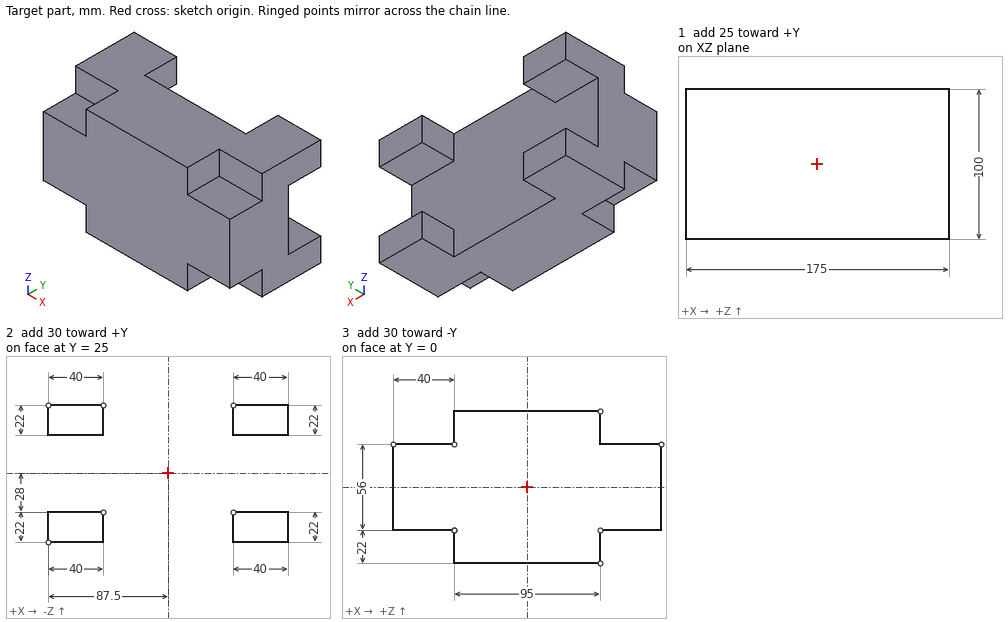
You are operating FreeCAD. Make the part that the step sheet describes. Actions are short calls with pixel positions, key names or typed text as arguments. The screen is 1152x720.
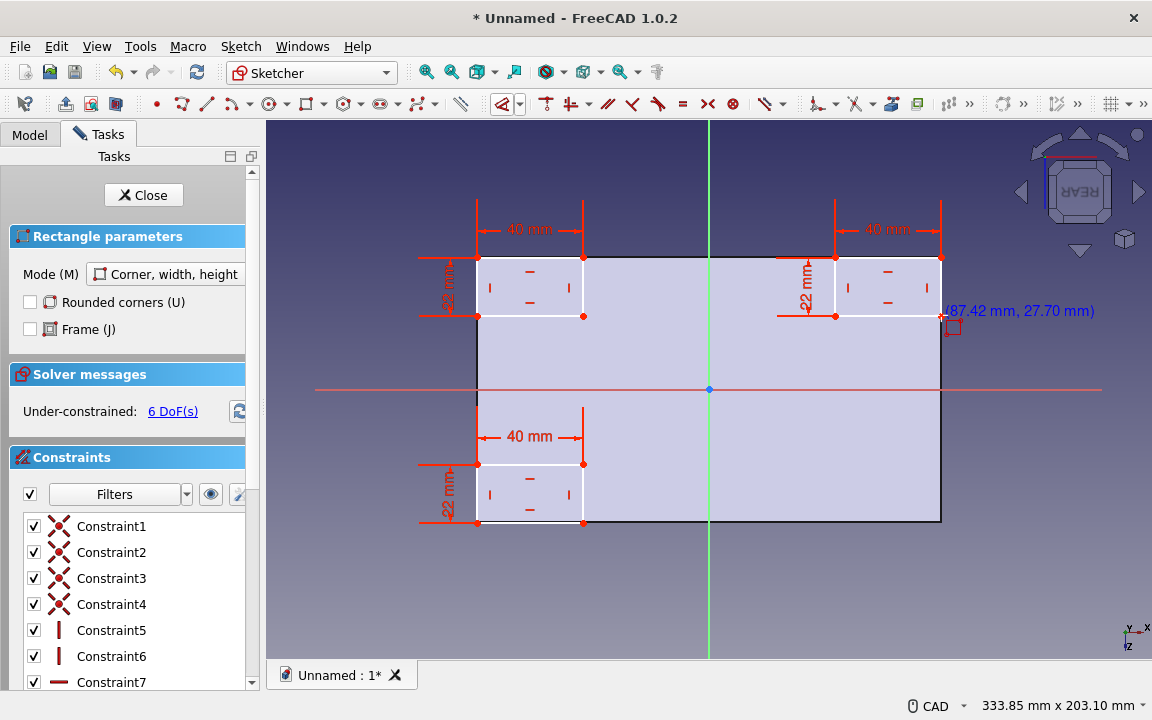
click(835, 464)
move(941, 522)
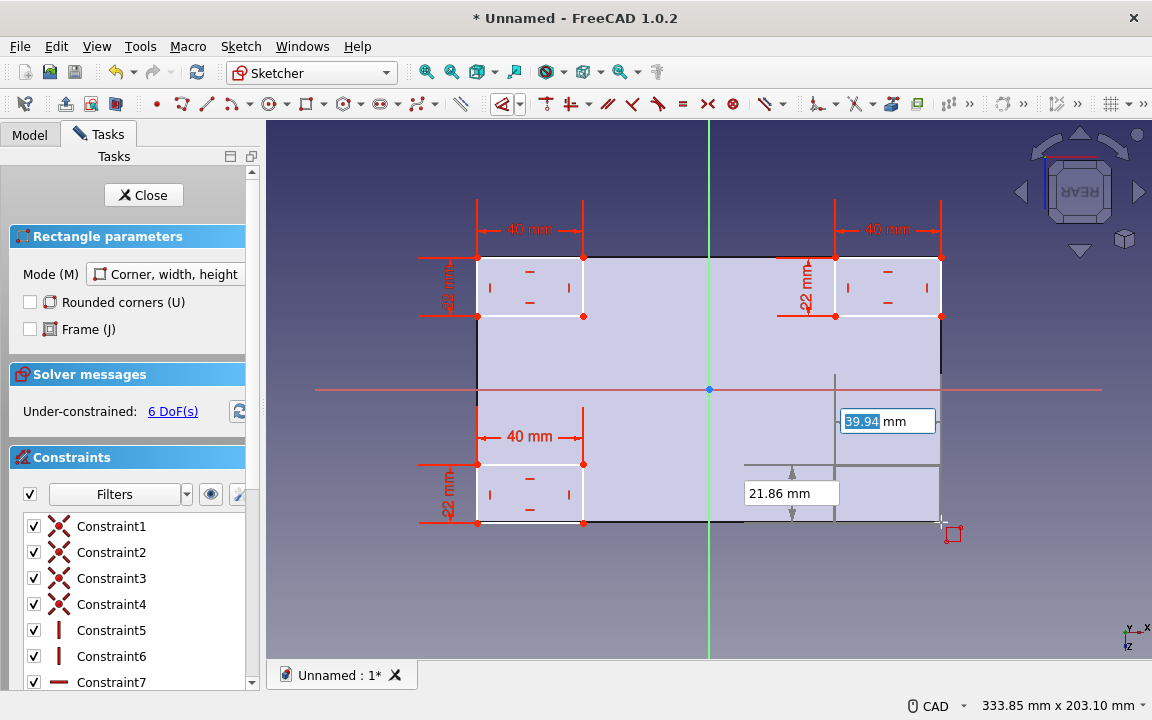
text(40)
key(Tab)
text(22)
key(Return)
key(Escape)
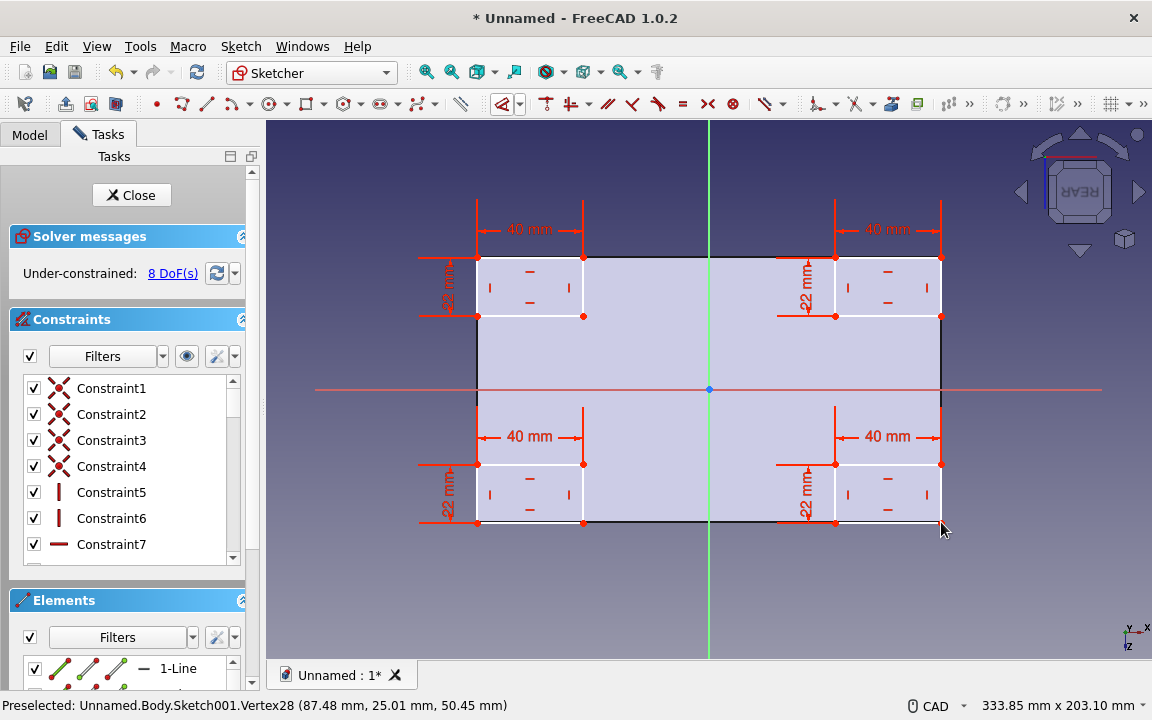
click(477, 523)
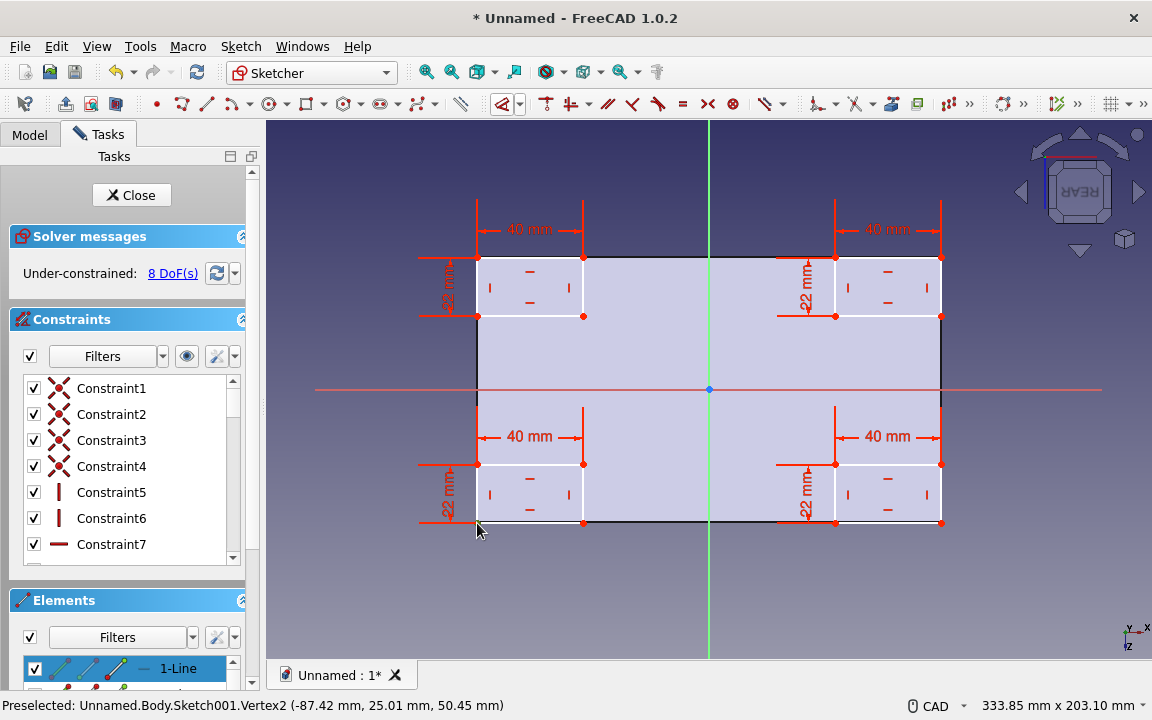
click(477, 258)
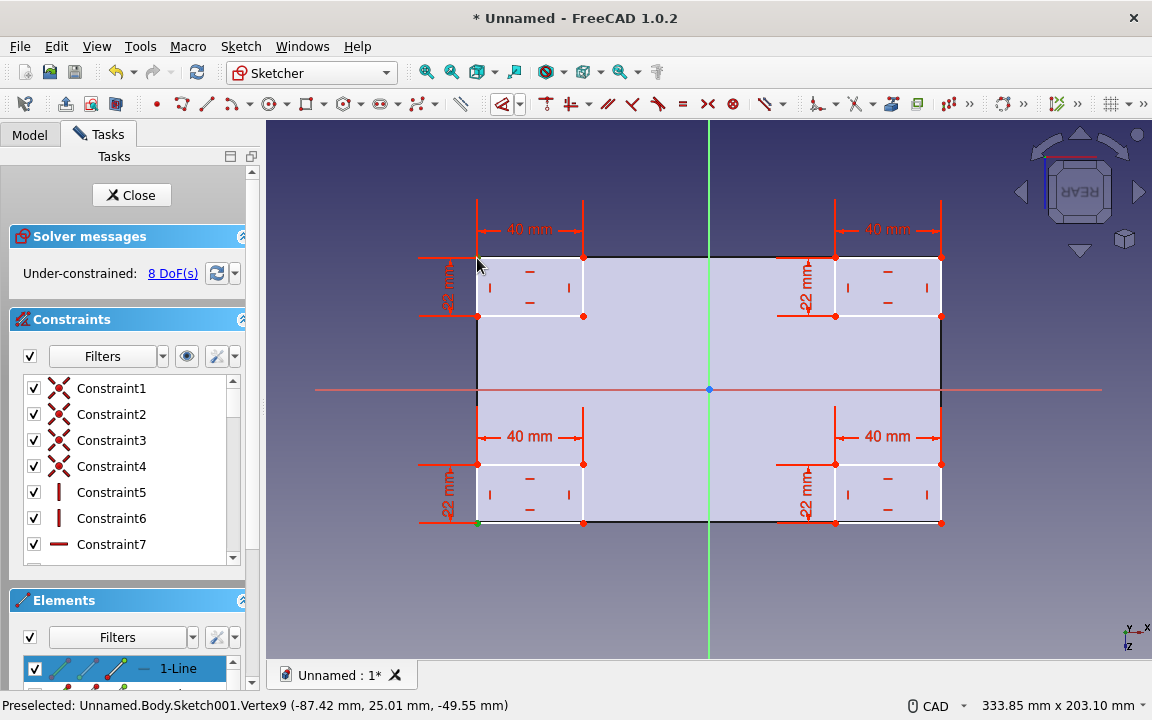
click(343, 390)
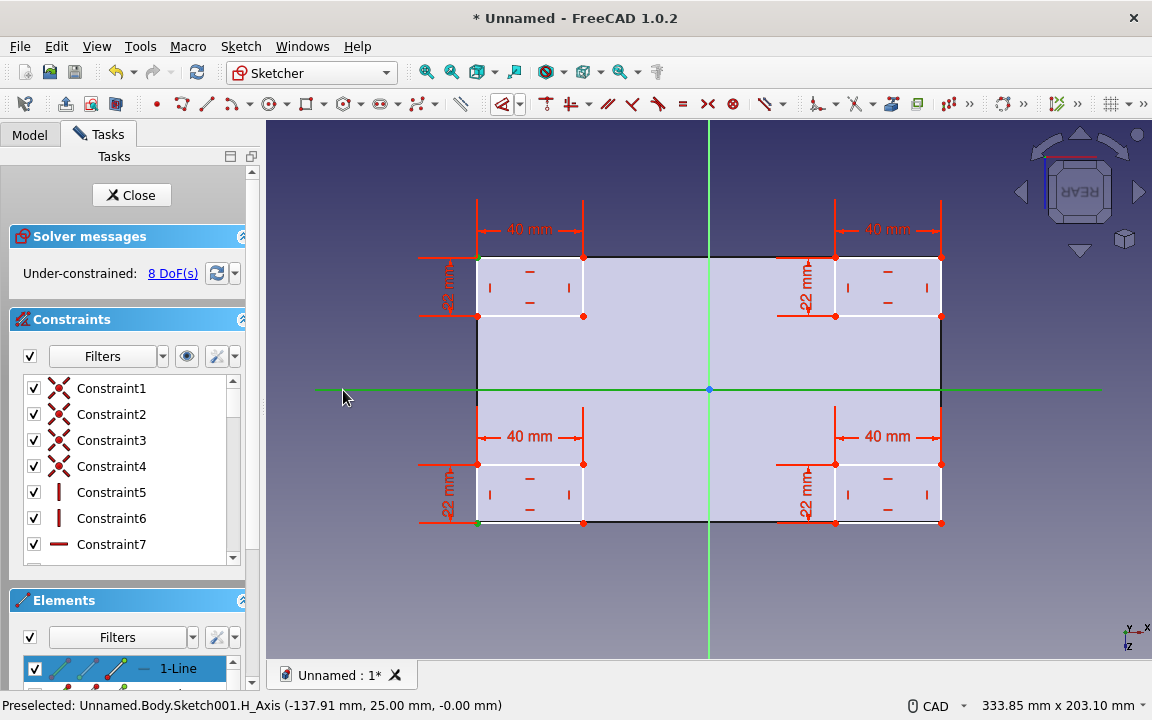
click(708, 104)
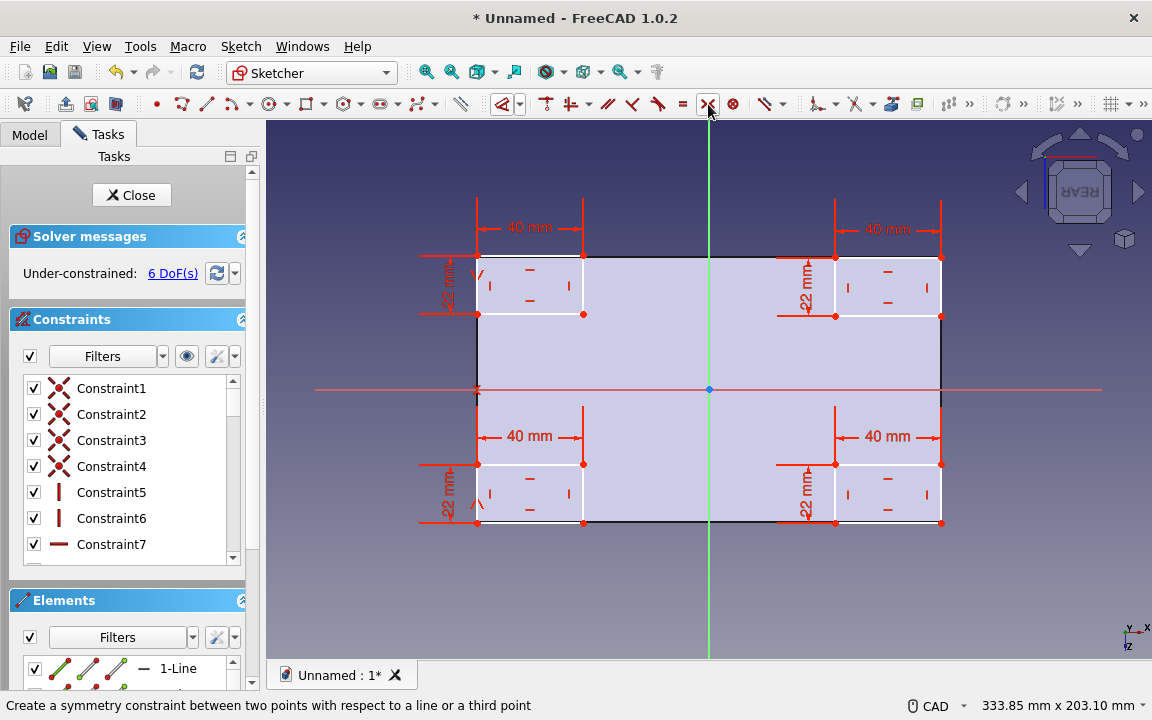
click(583, 256)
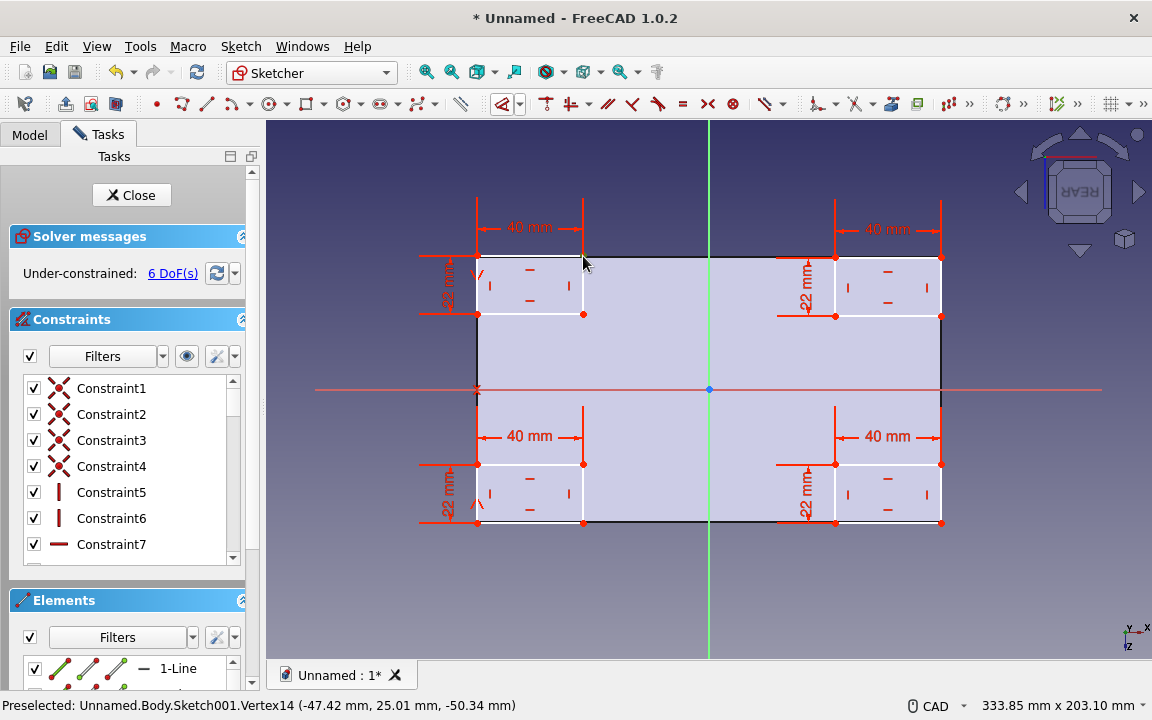
click(835, 258)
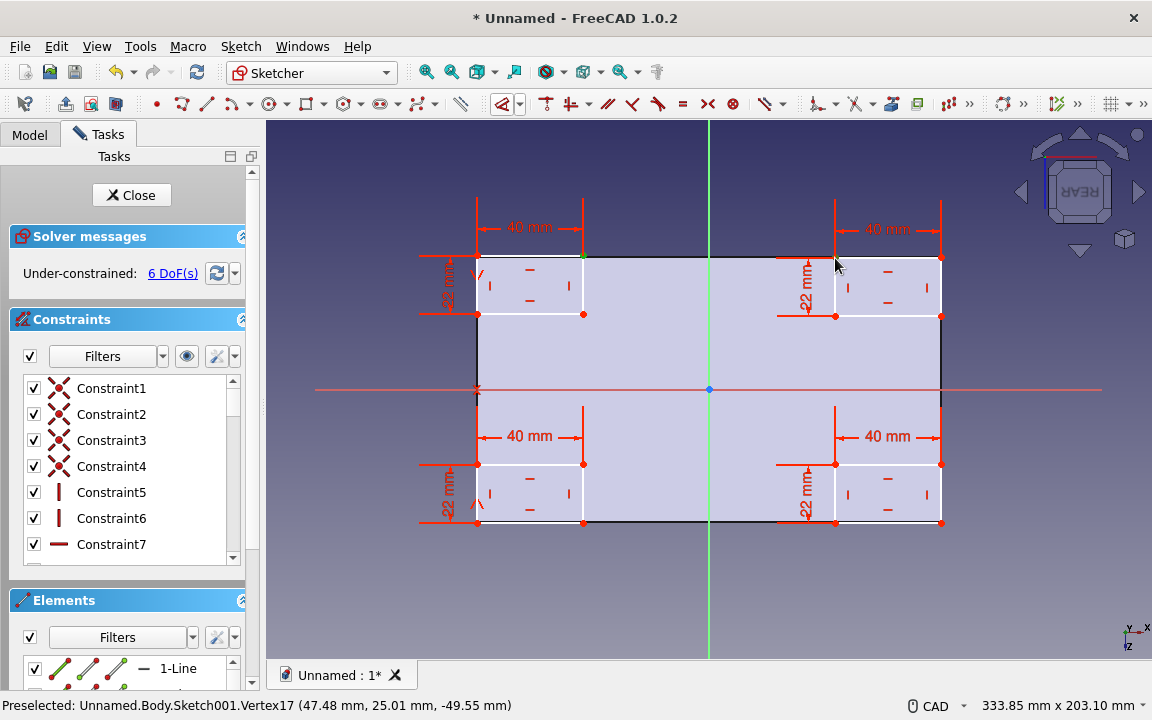
click(709, 596)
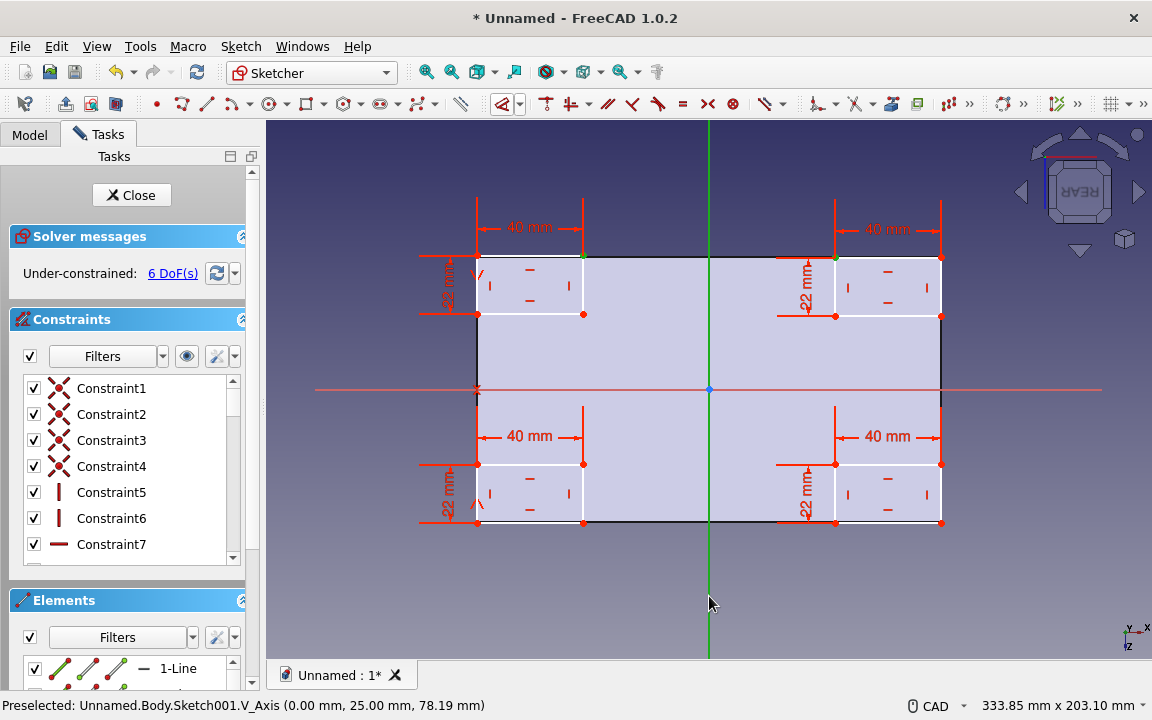
click(708, 104)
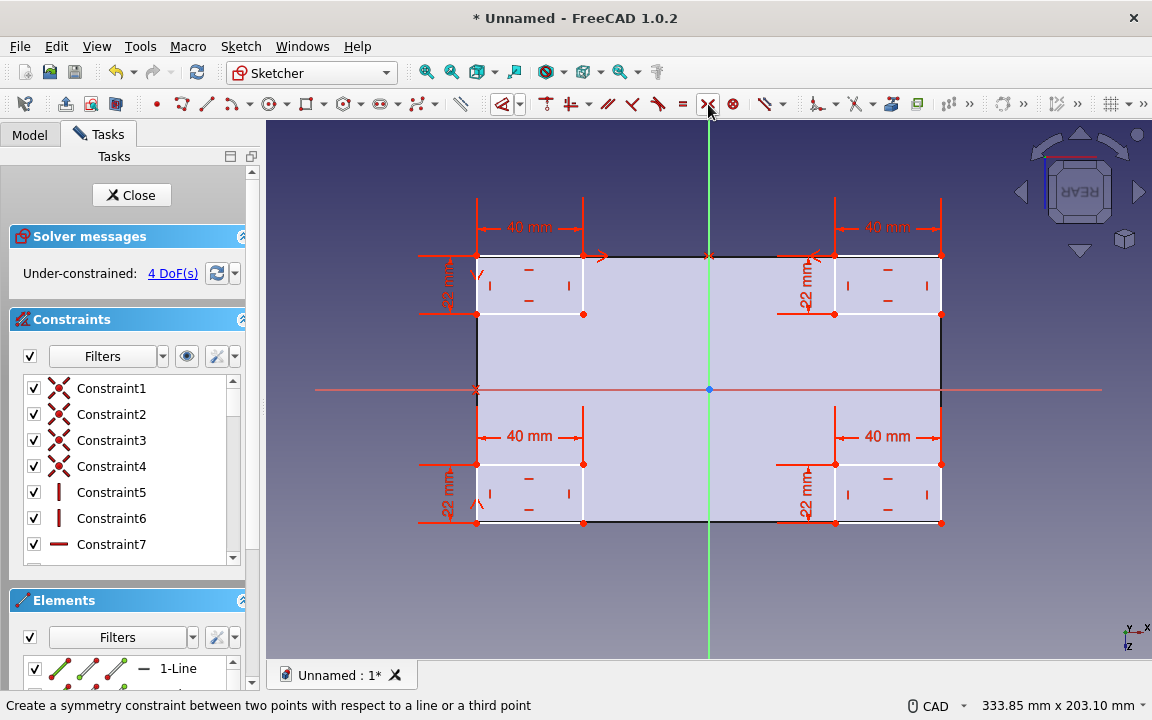
click(583, 465)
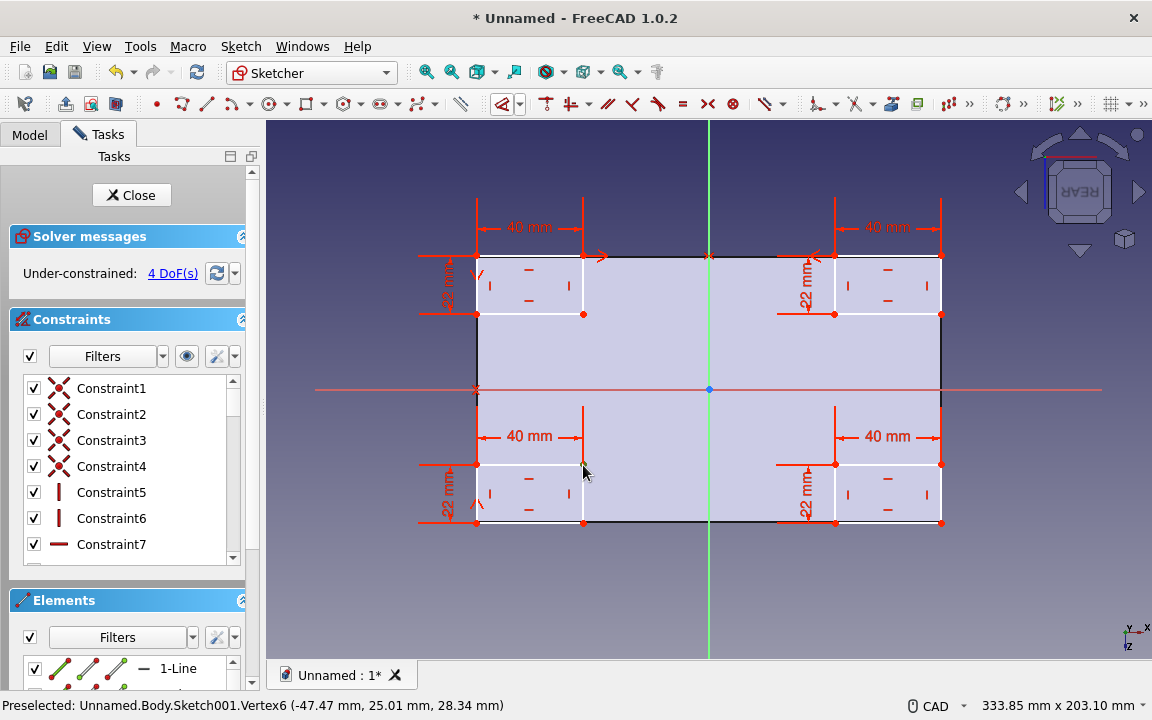
click(835, 465)